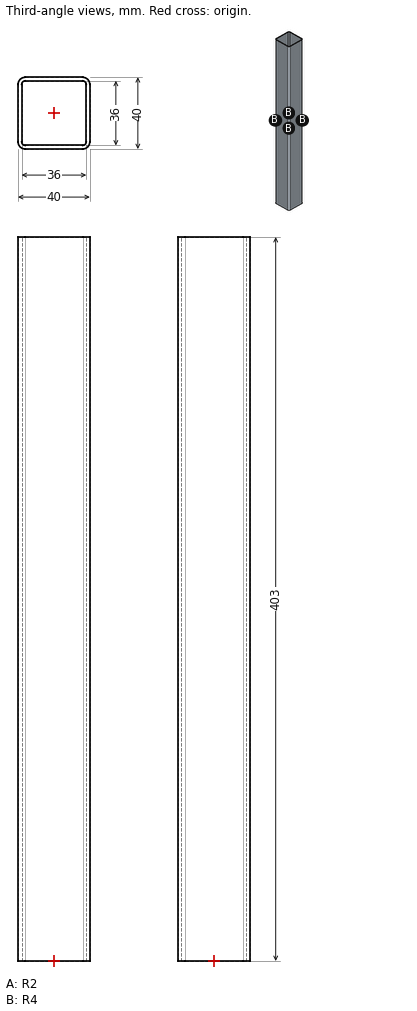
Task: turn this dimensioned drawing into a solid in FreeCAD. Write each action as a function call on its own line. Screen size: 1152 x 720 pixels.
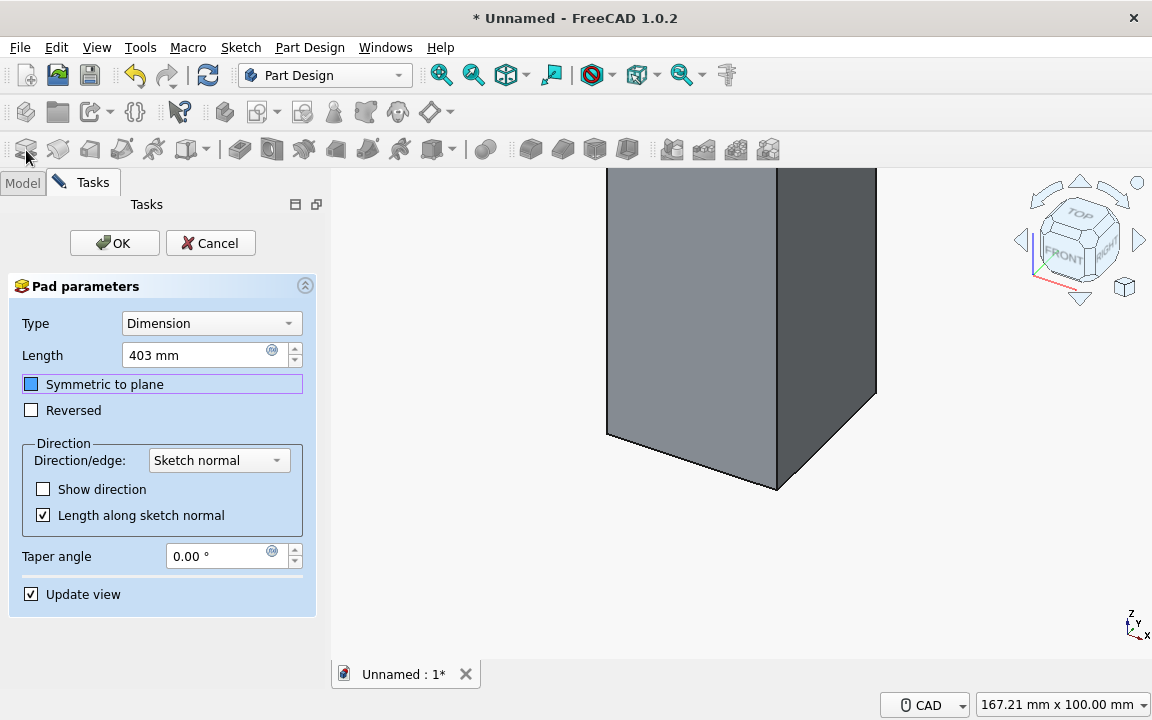
click(115, 243)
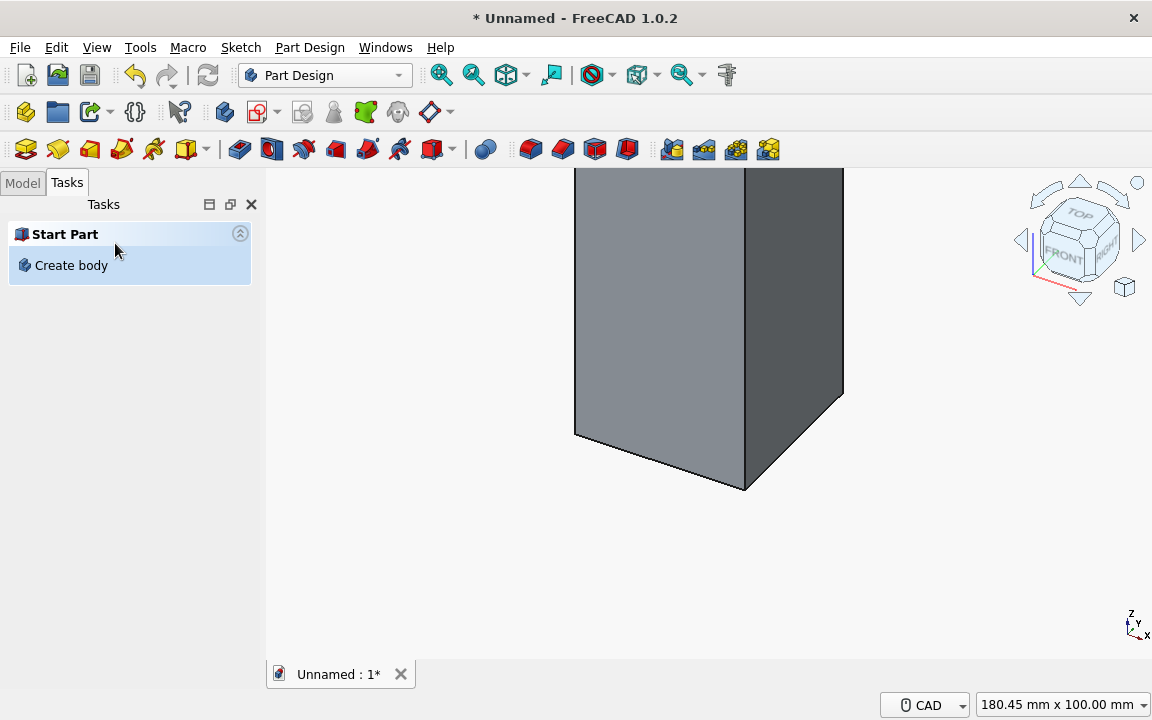
click(442, 76)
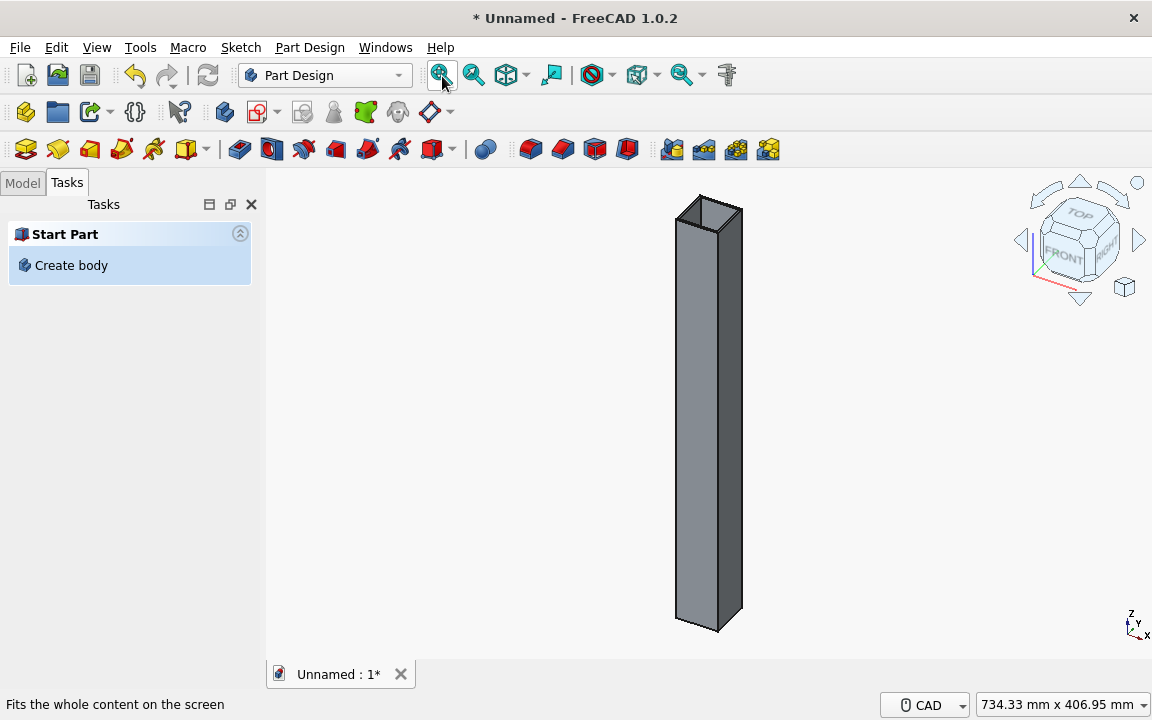
key(0)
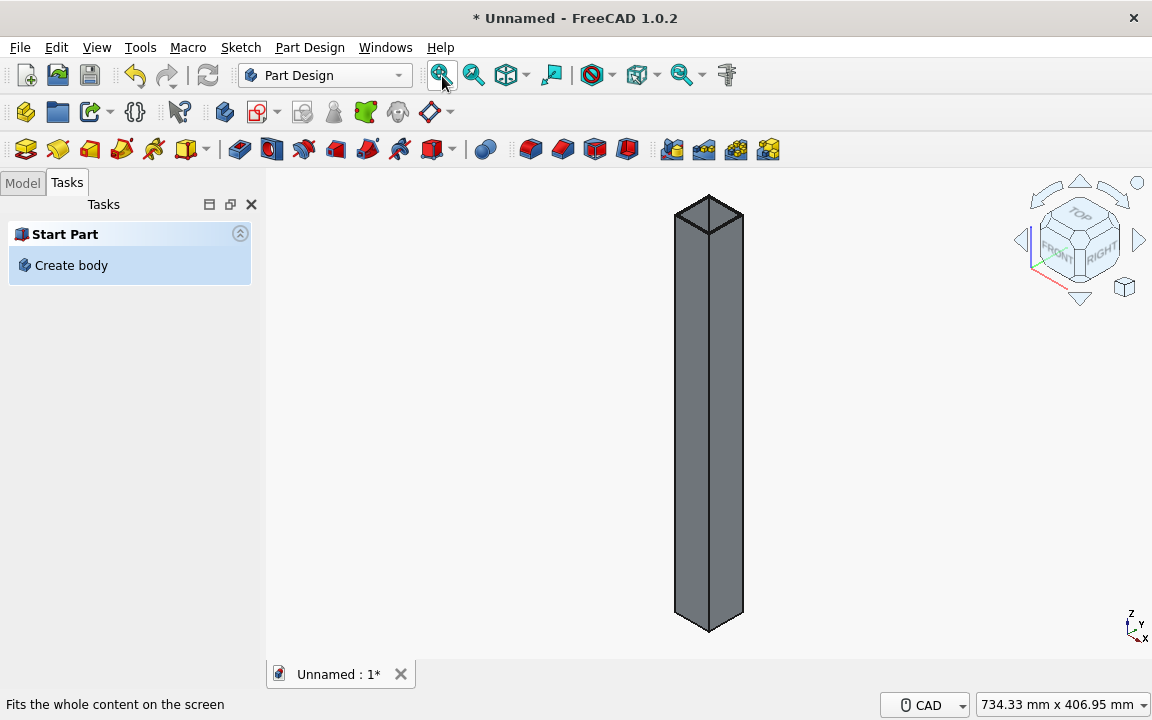
key(2)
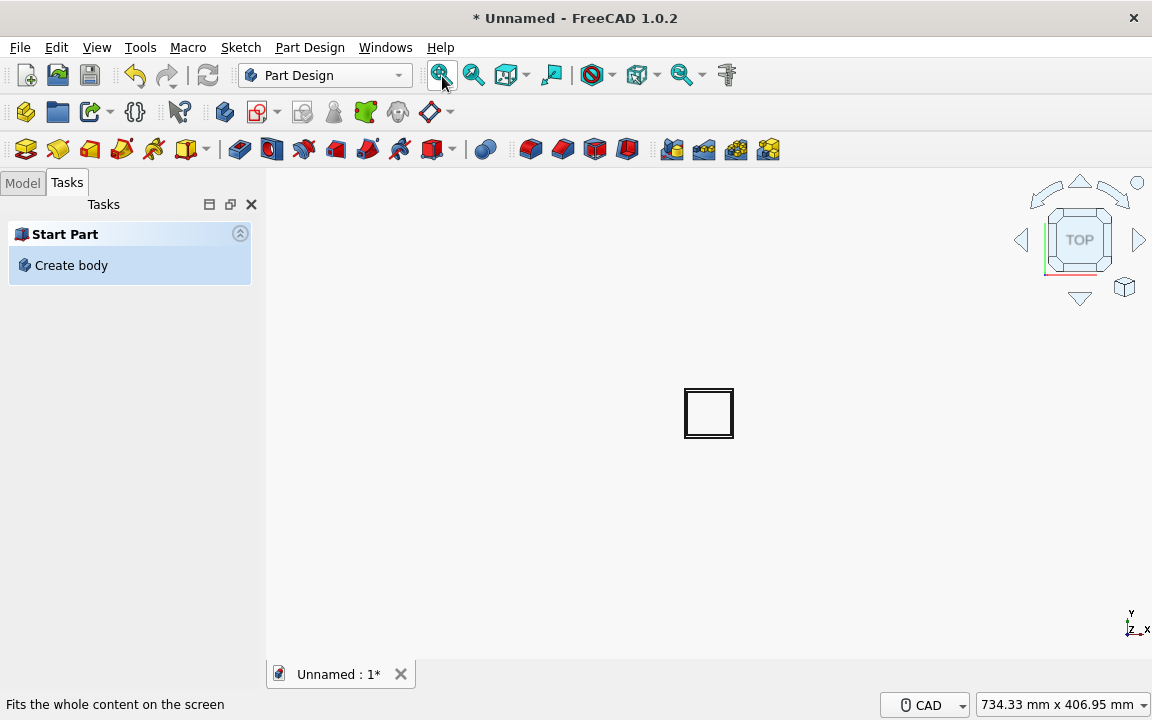
click(442, 76)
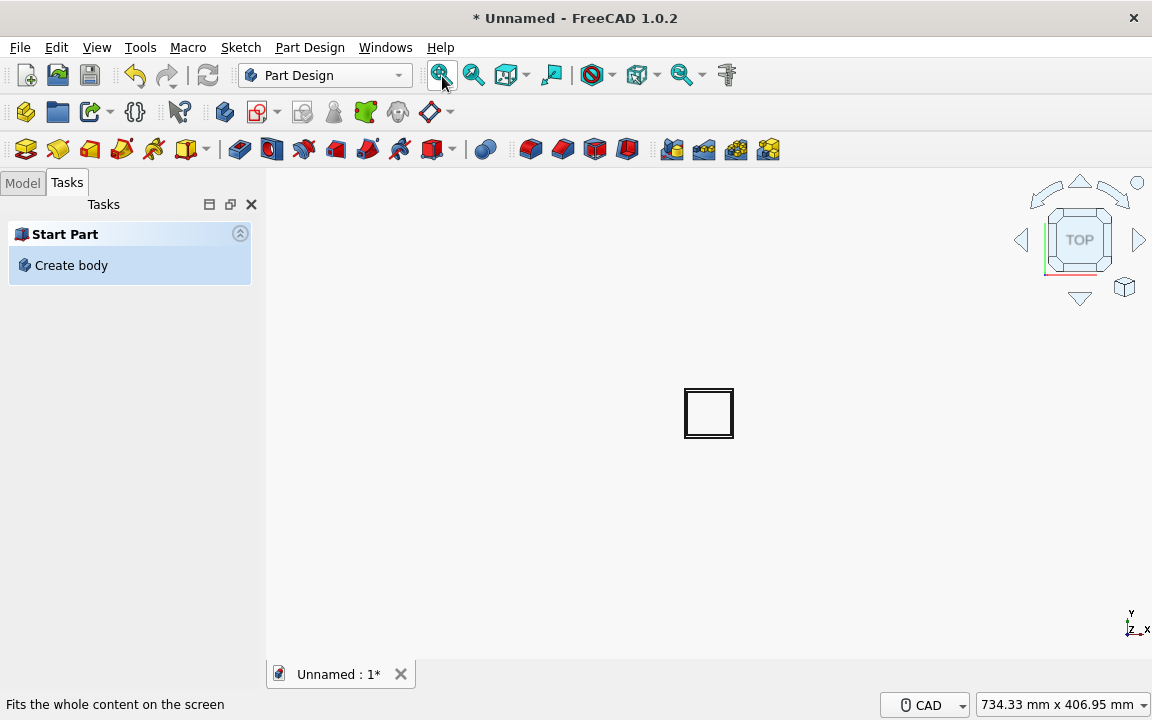
key(1)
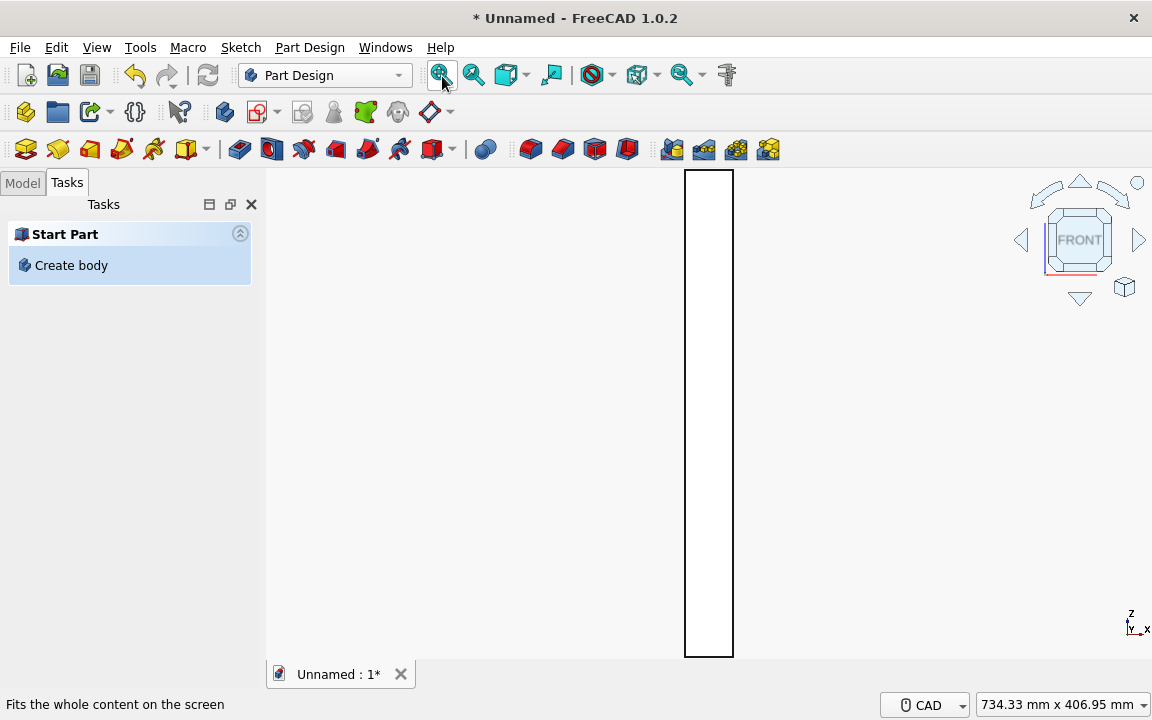
key(3)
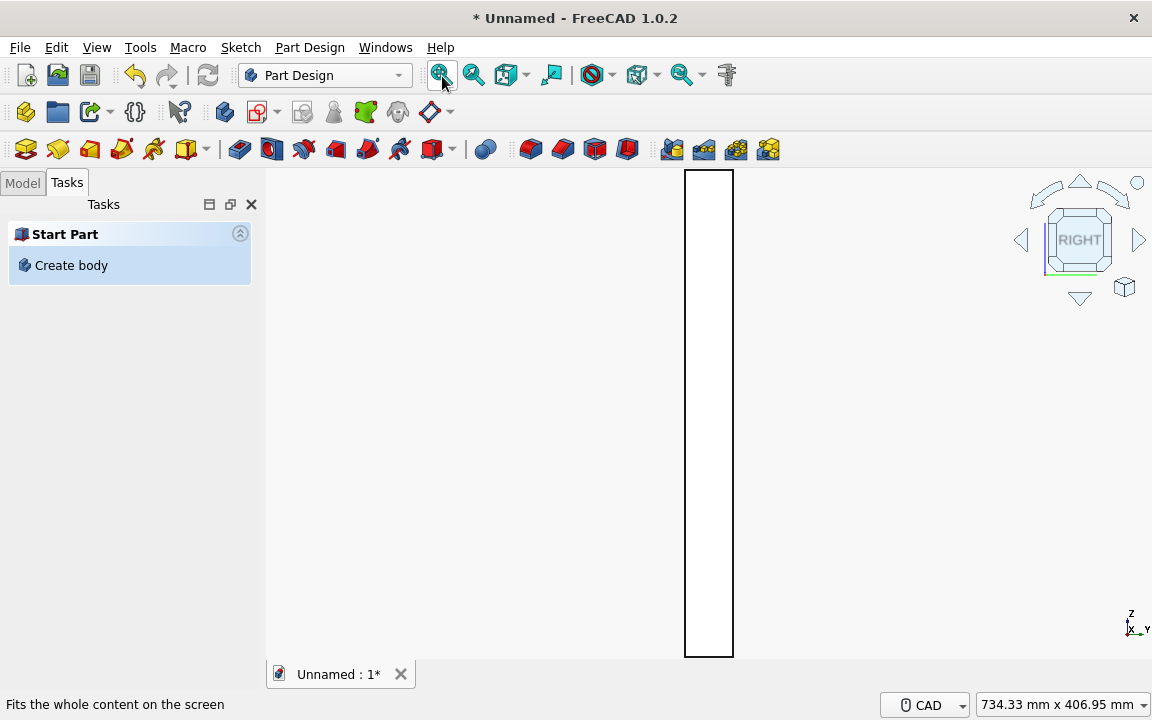
key(5)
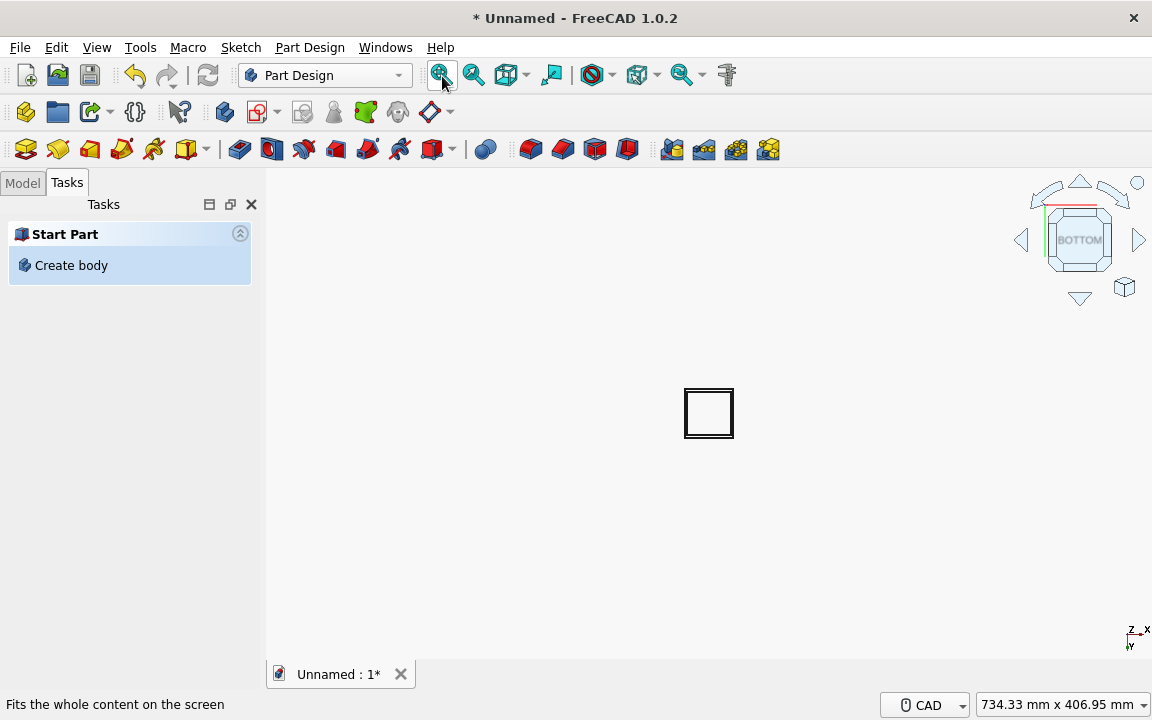
click(442, 76)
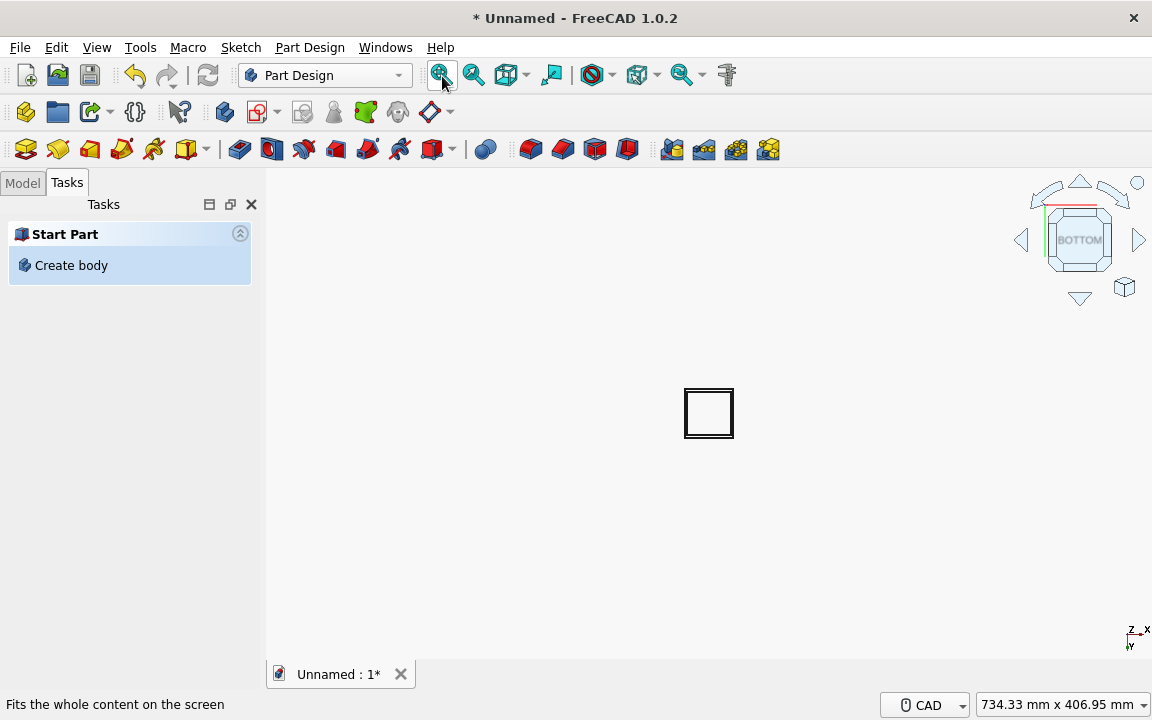
key(4)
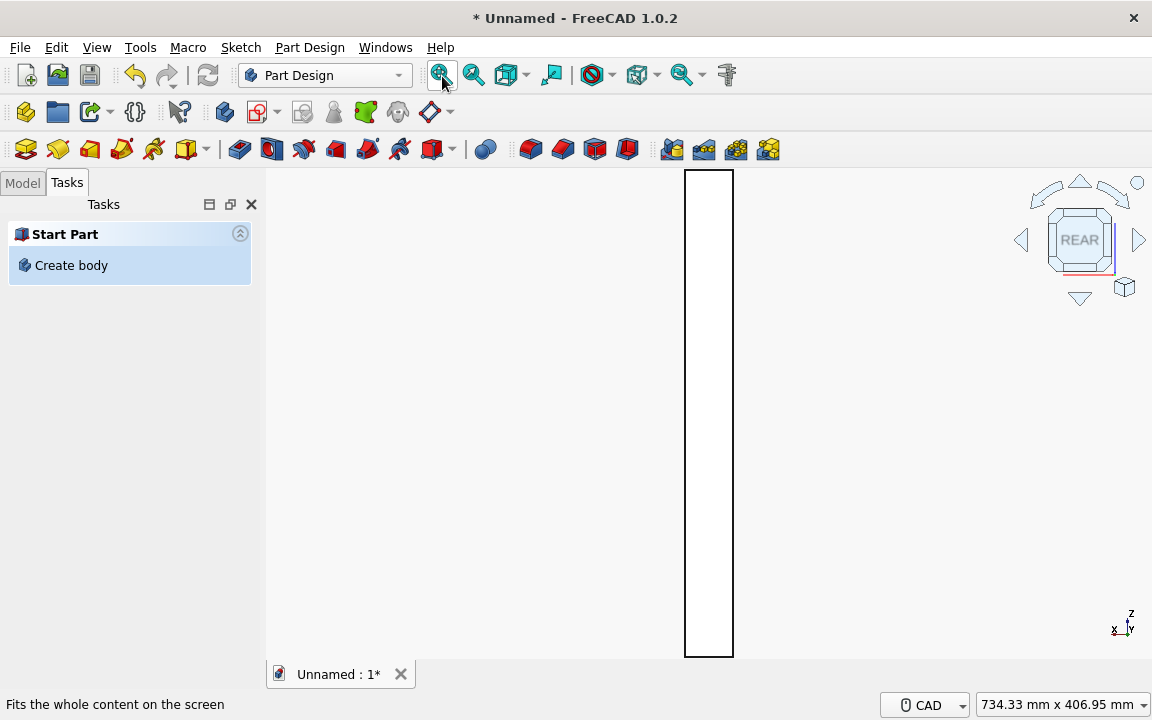
key(6)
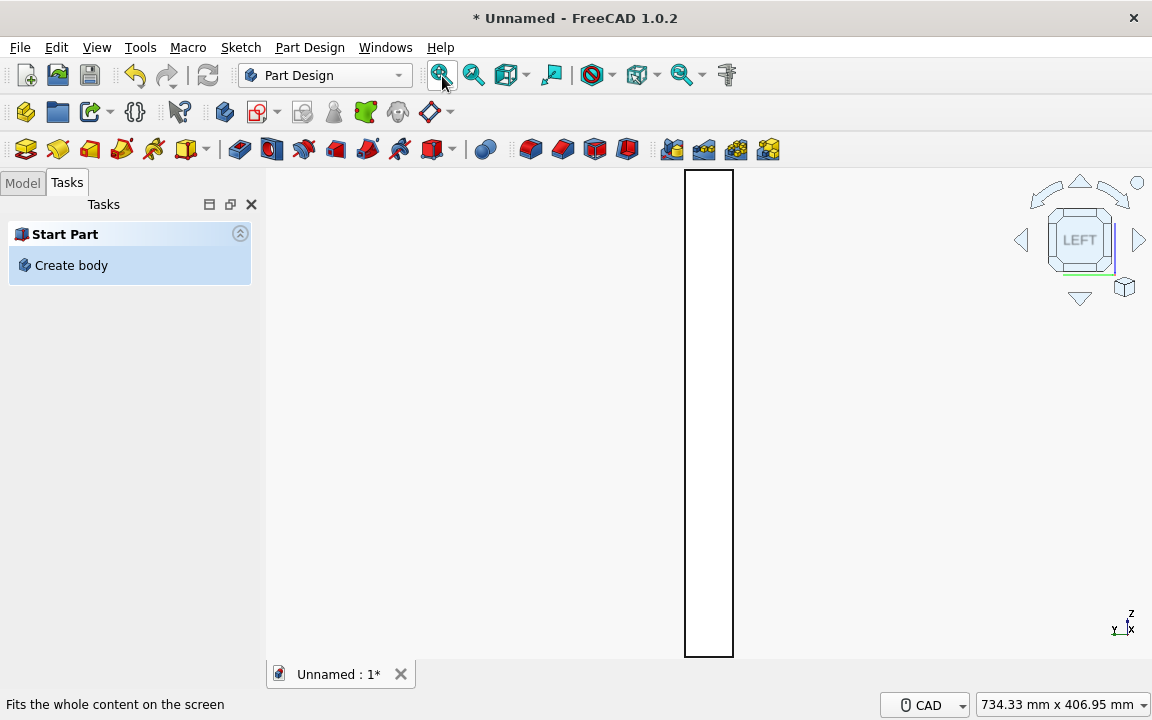
key(v)
key(3)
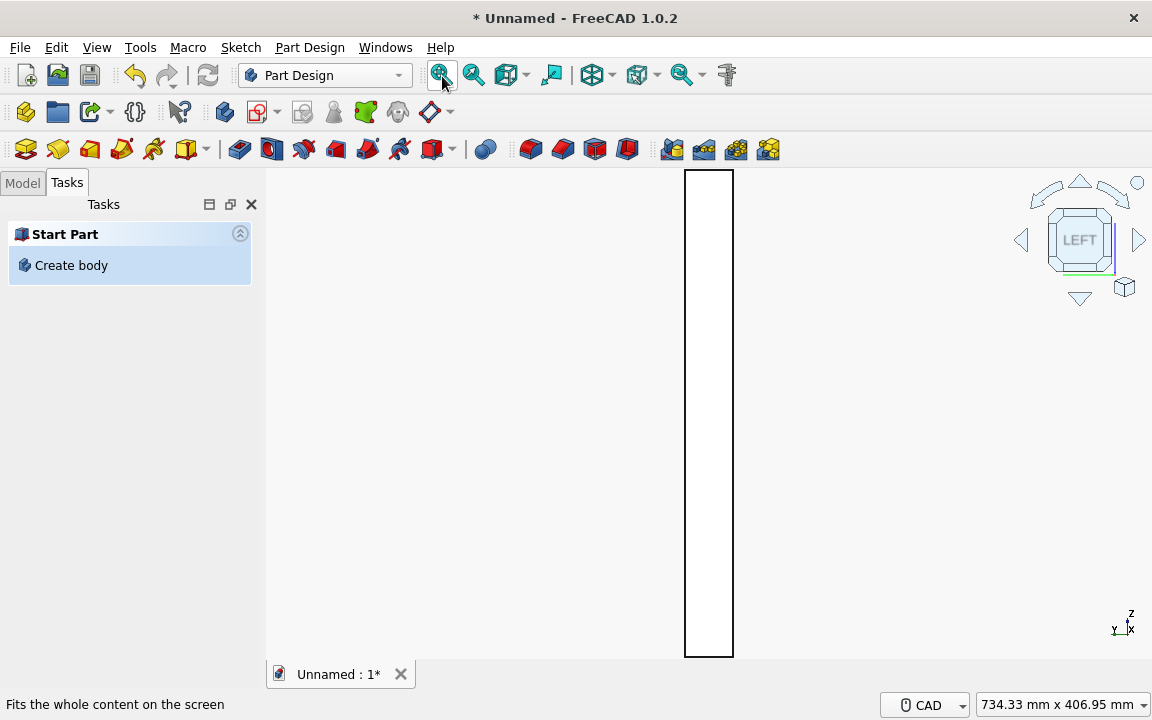
key(0)